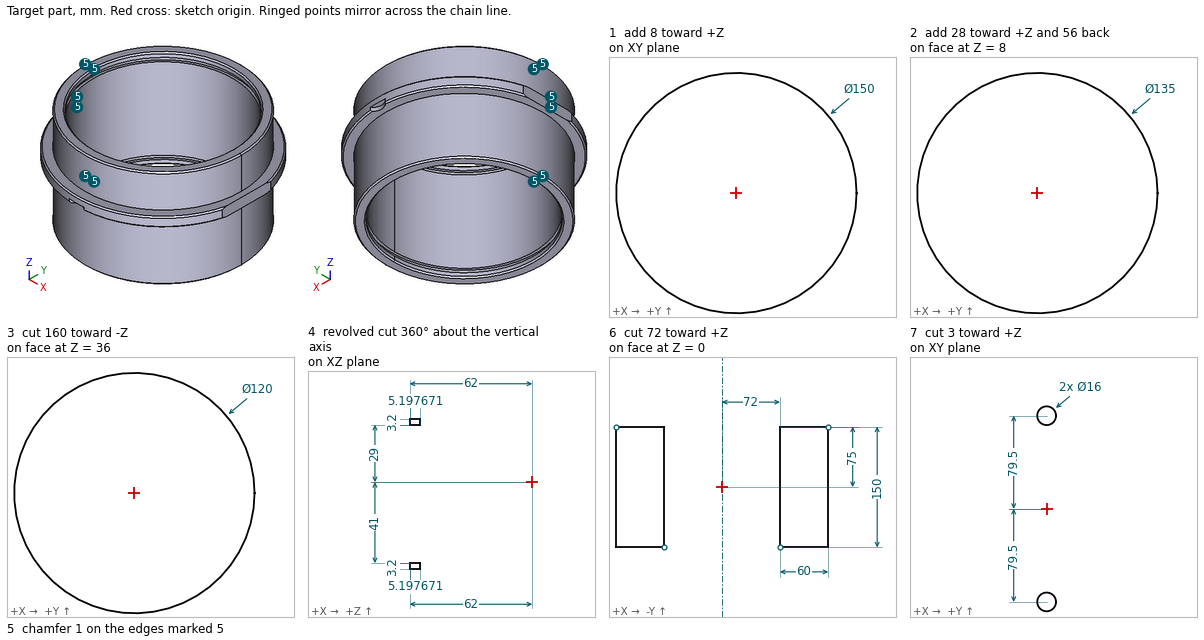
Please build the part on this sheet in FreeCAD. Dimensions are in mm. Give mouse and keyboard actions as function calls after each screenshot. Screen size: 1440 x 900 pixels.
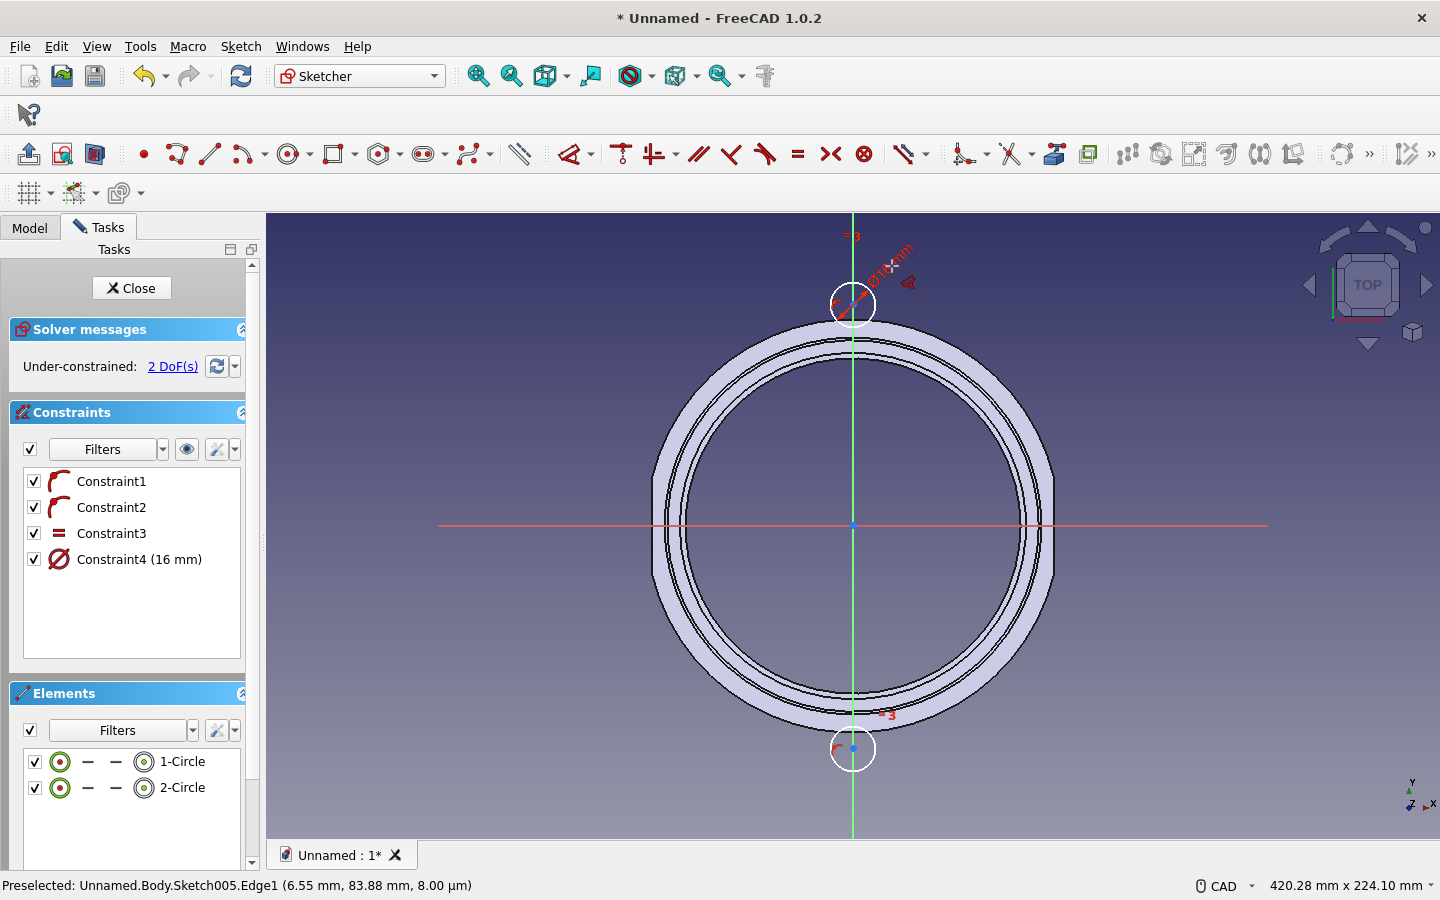
click(853, 305)
click(887, 415)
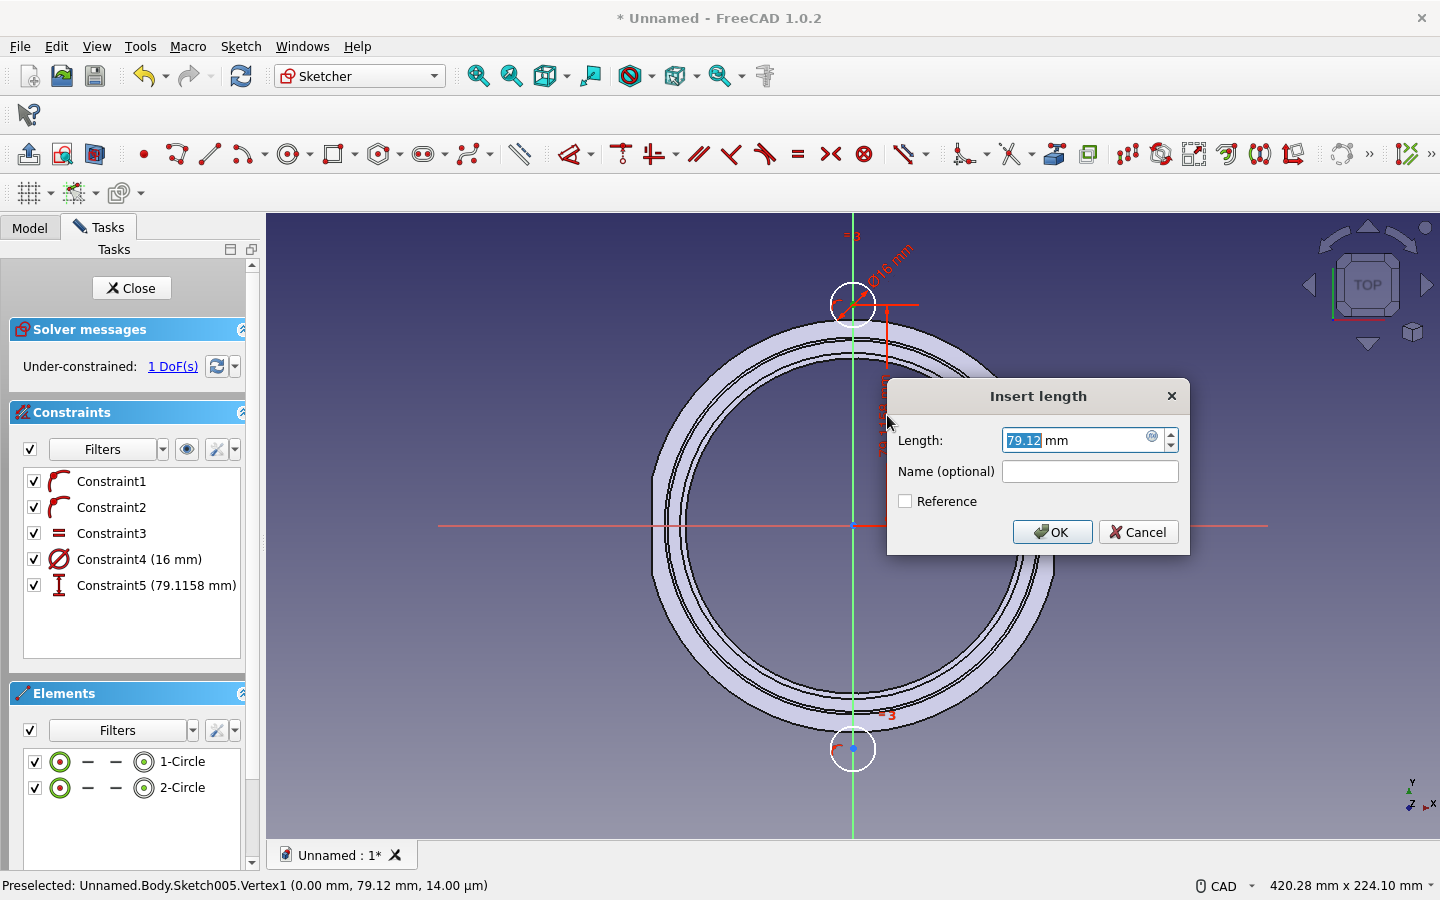
text(79.5)
key(Return)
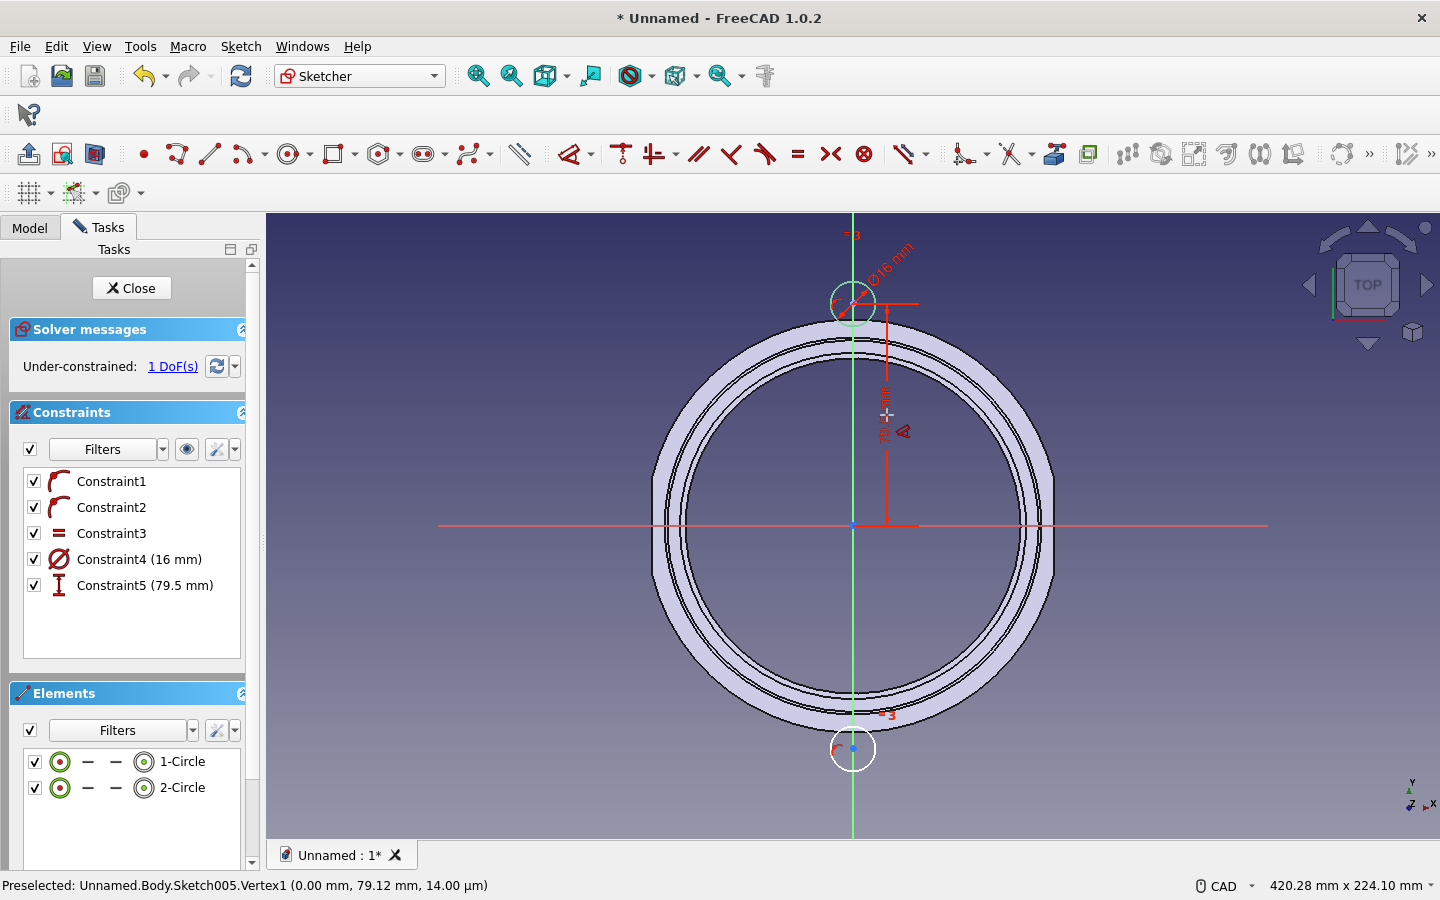
click(853, 749)
click(887, 638)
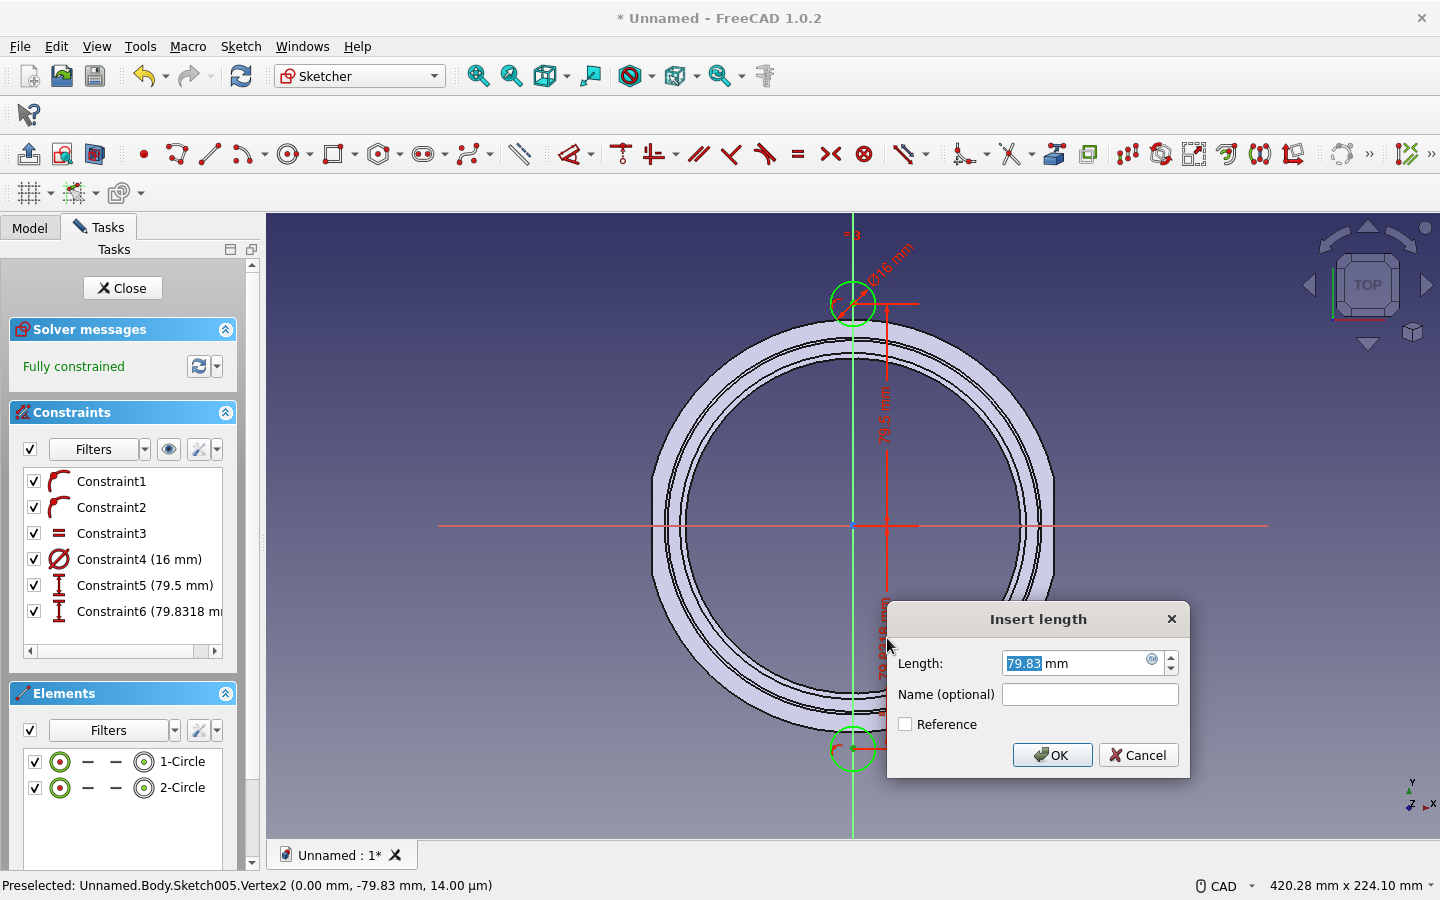
text(79.5)
key(Return)
key(Escape)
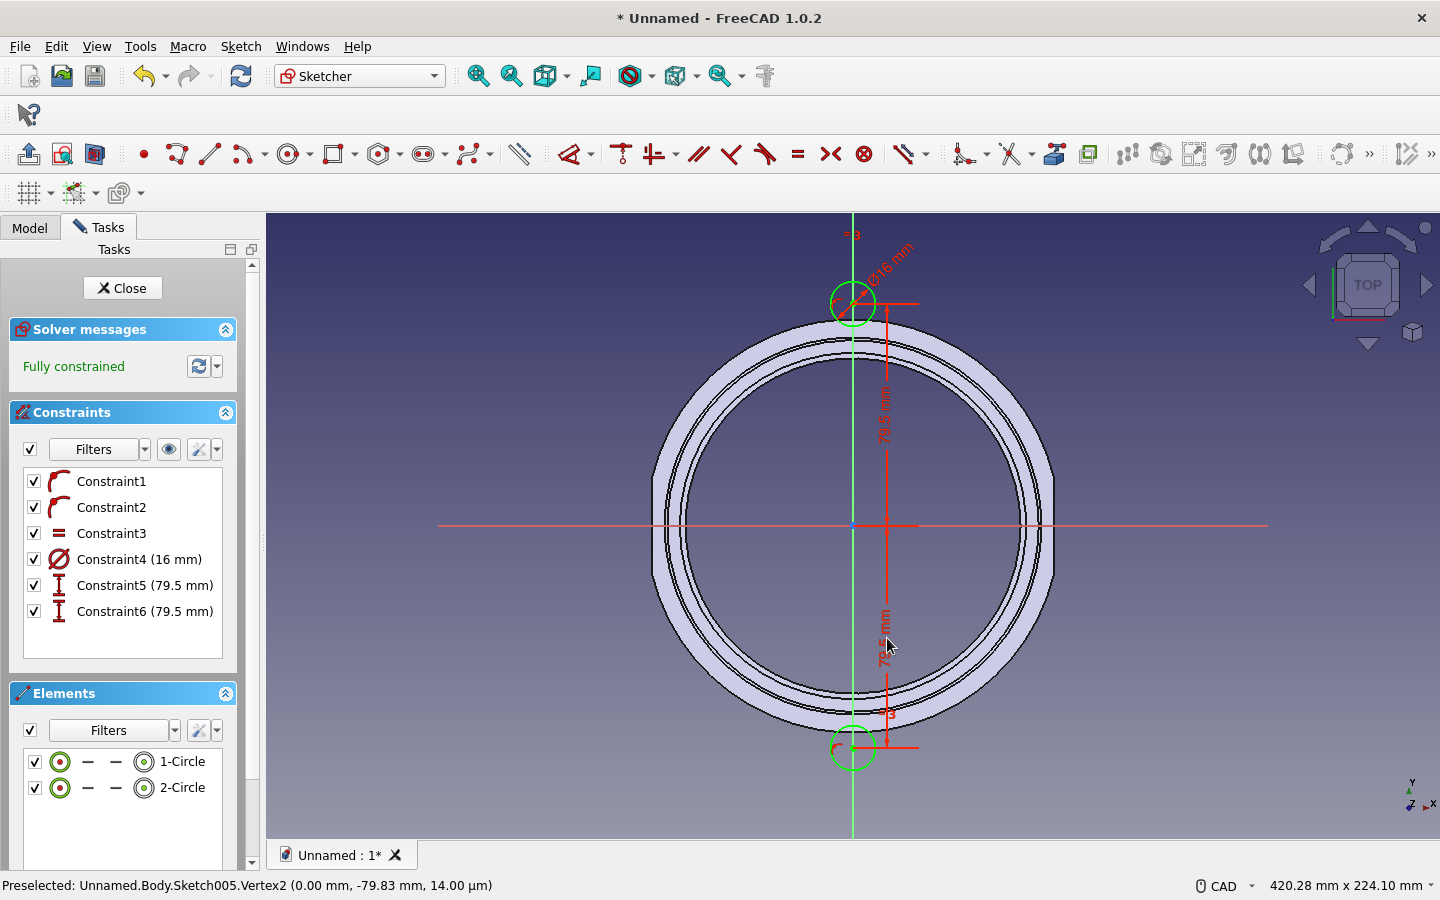
click(123, 288)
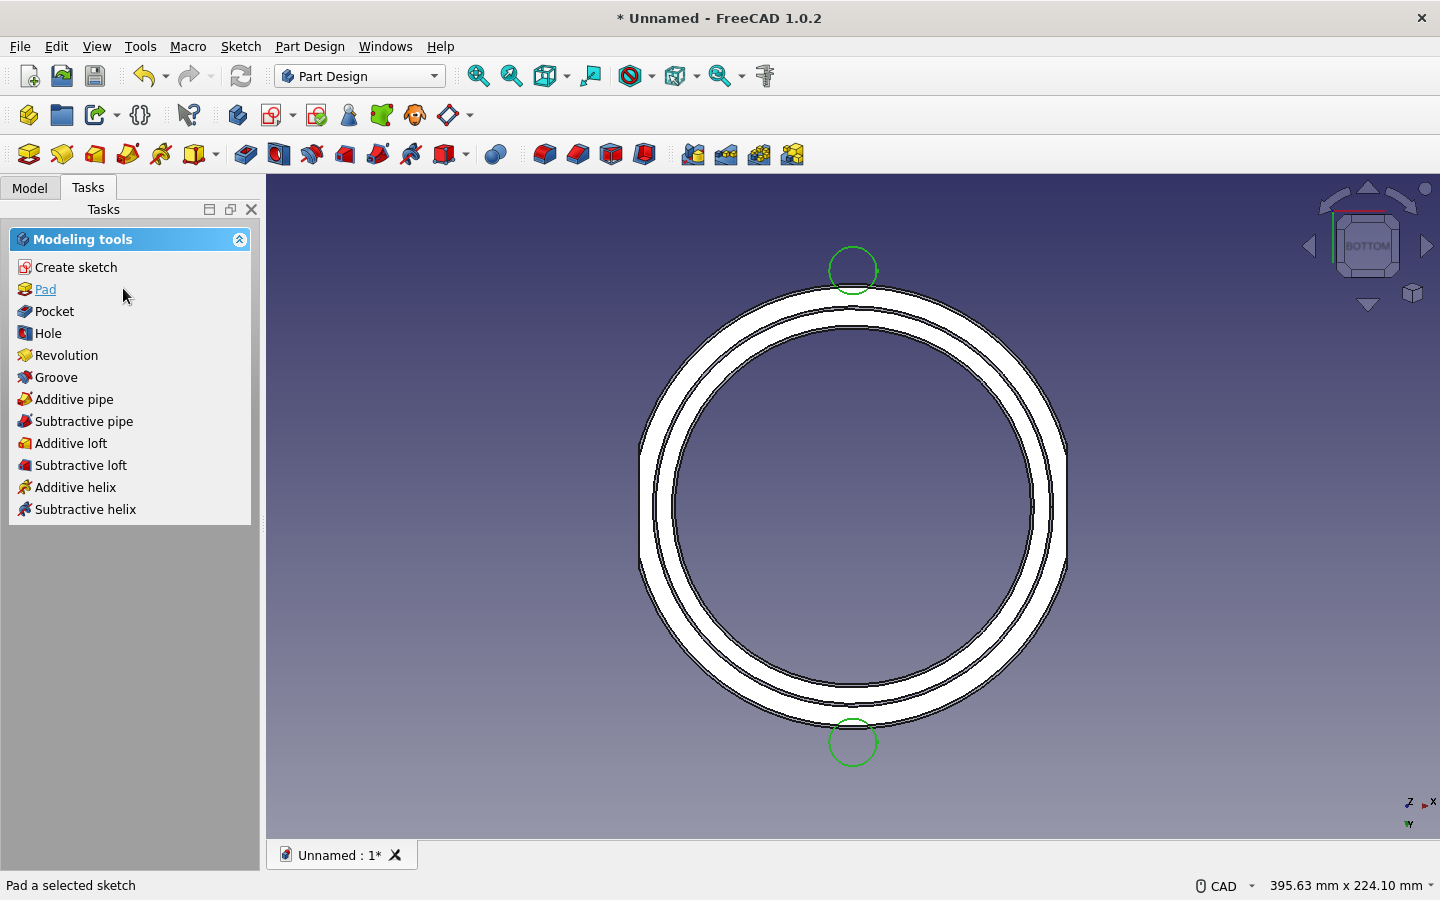
click(246, 154)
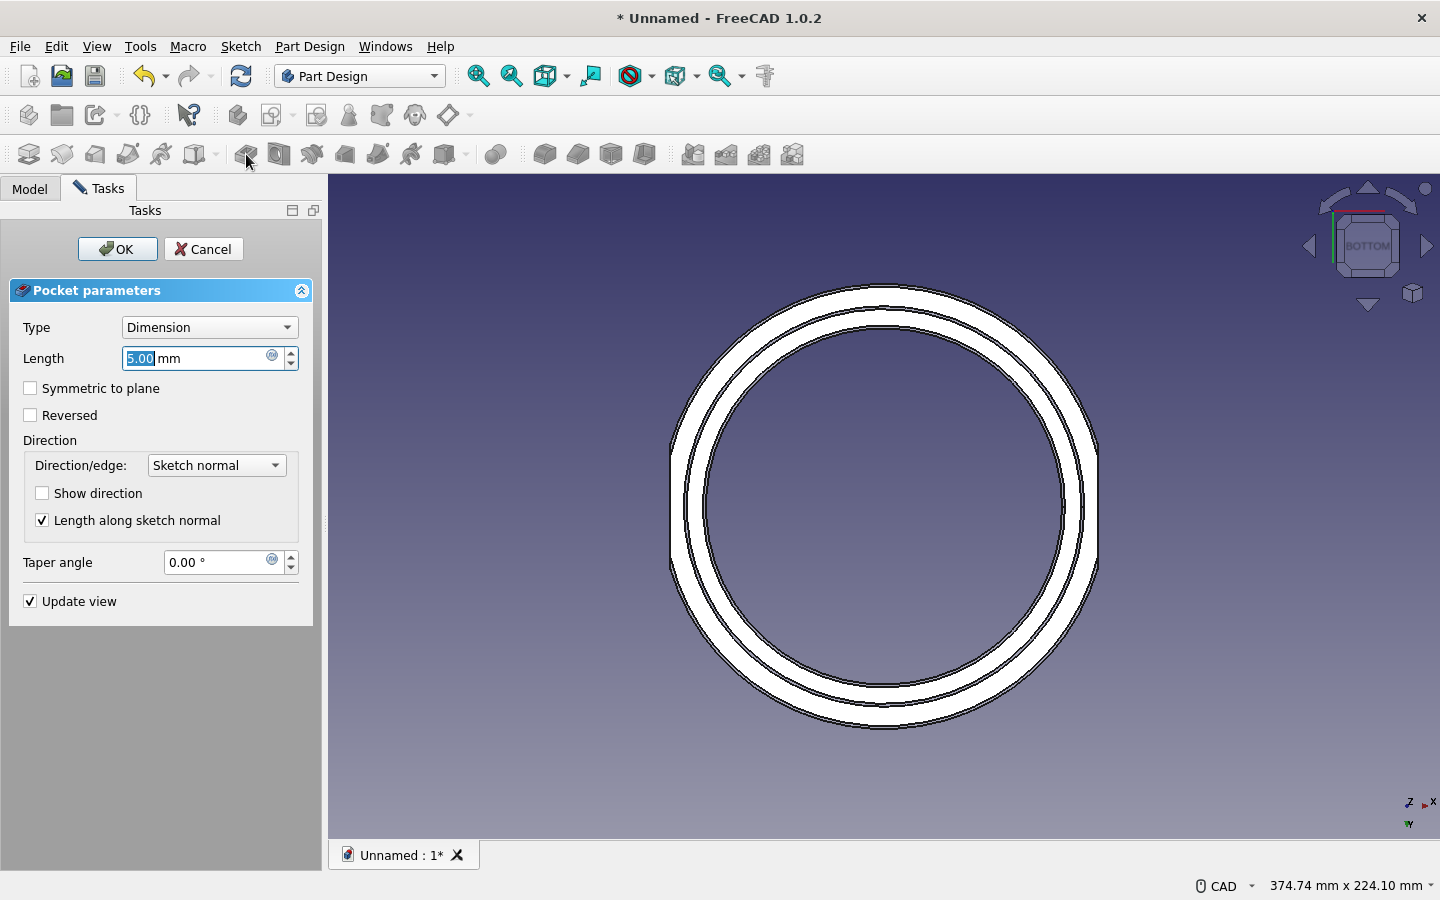
text(3)
key(Tab)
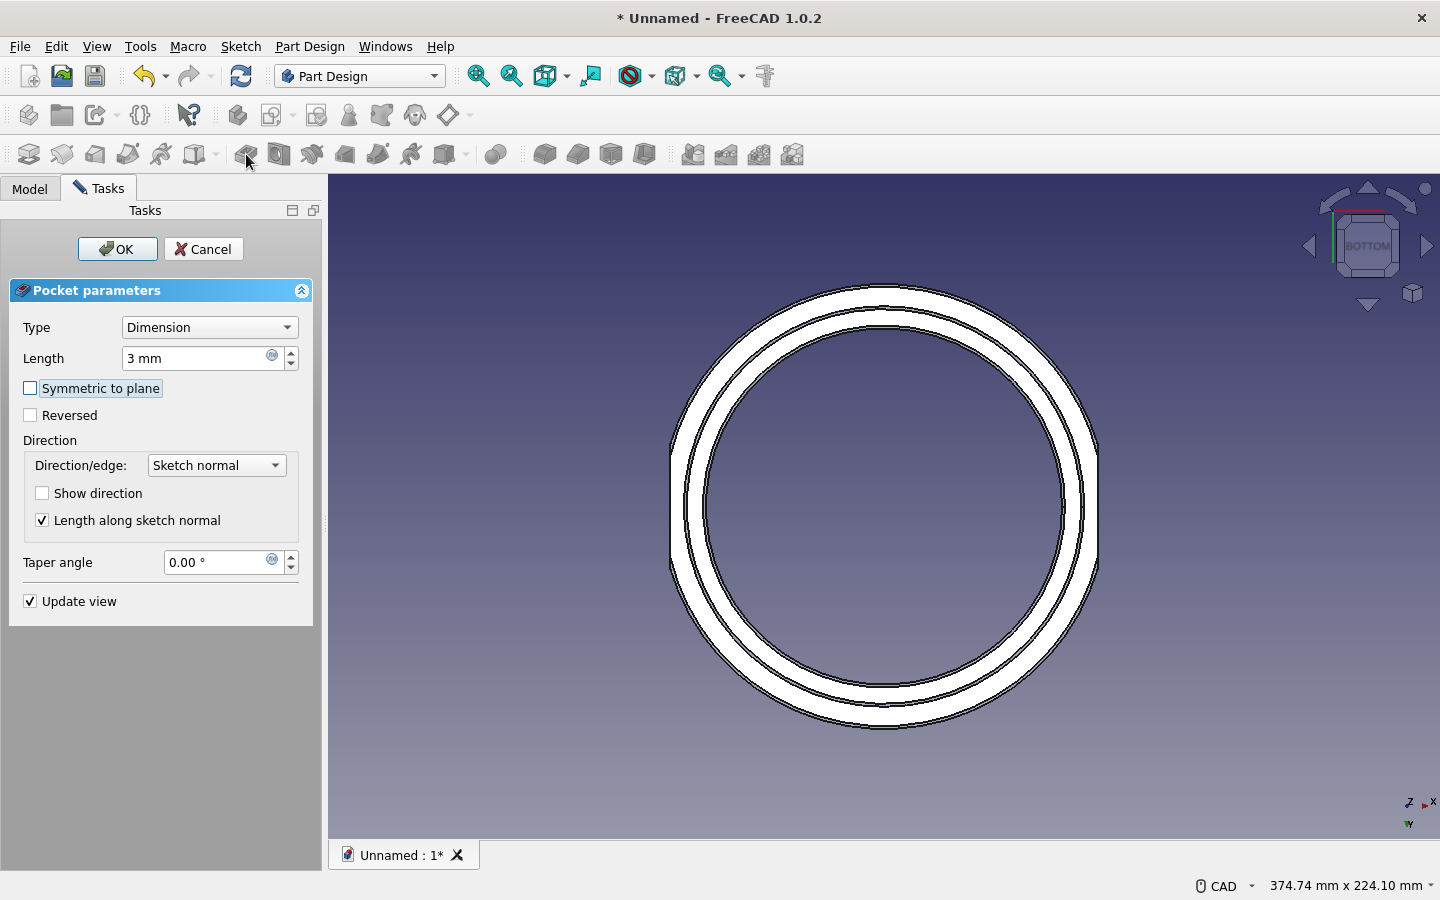
click(31, 415)